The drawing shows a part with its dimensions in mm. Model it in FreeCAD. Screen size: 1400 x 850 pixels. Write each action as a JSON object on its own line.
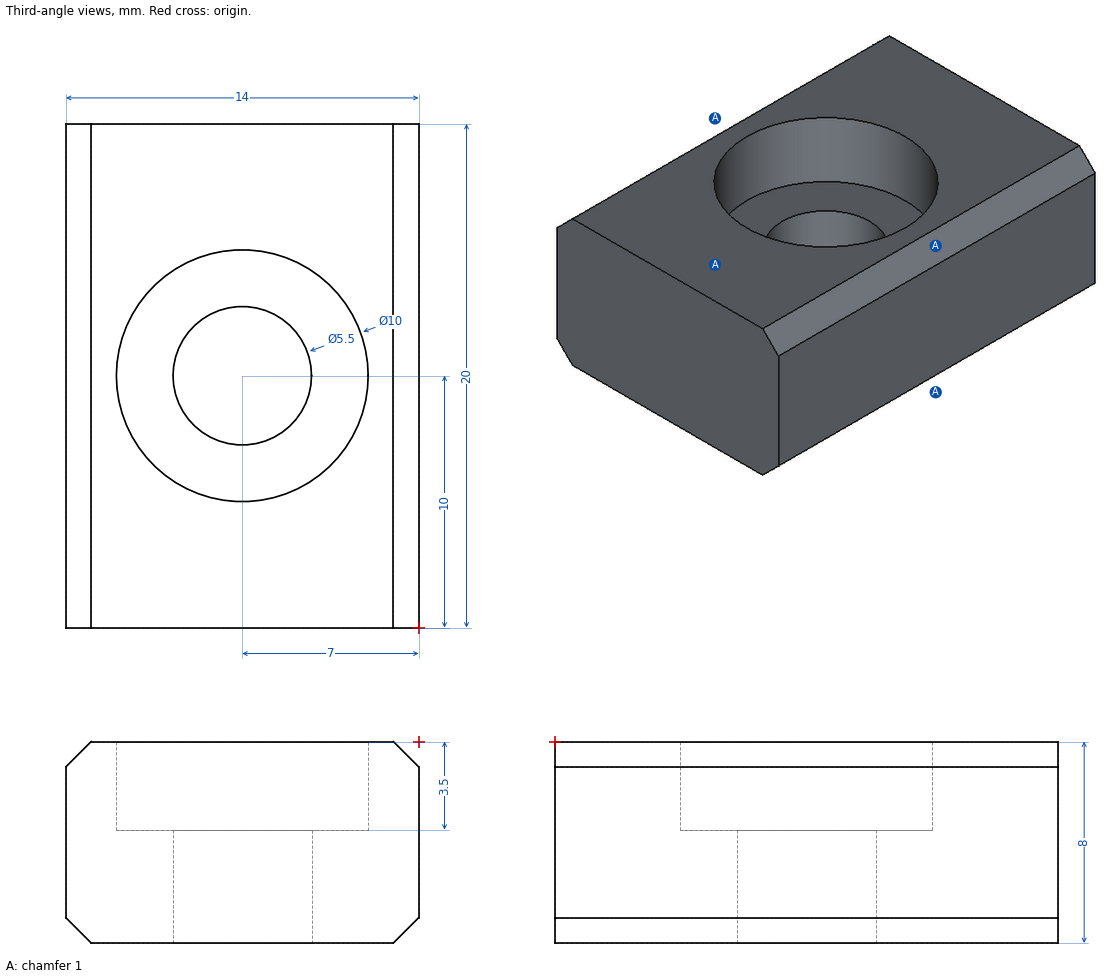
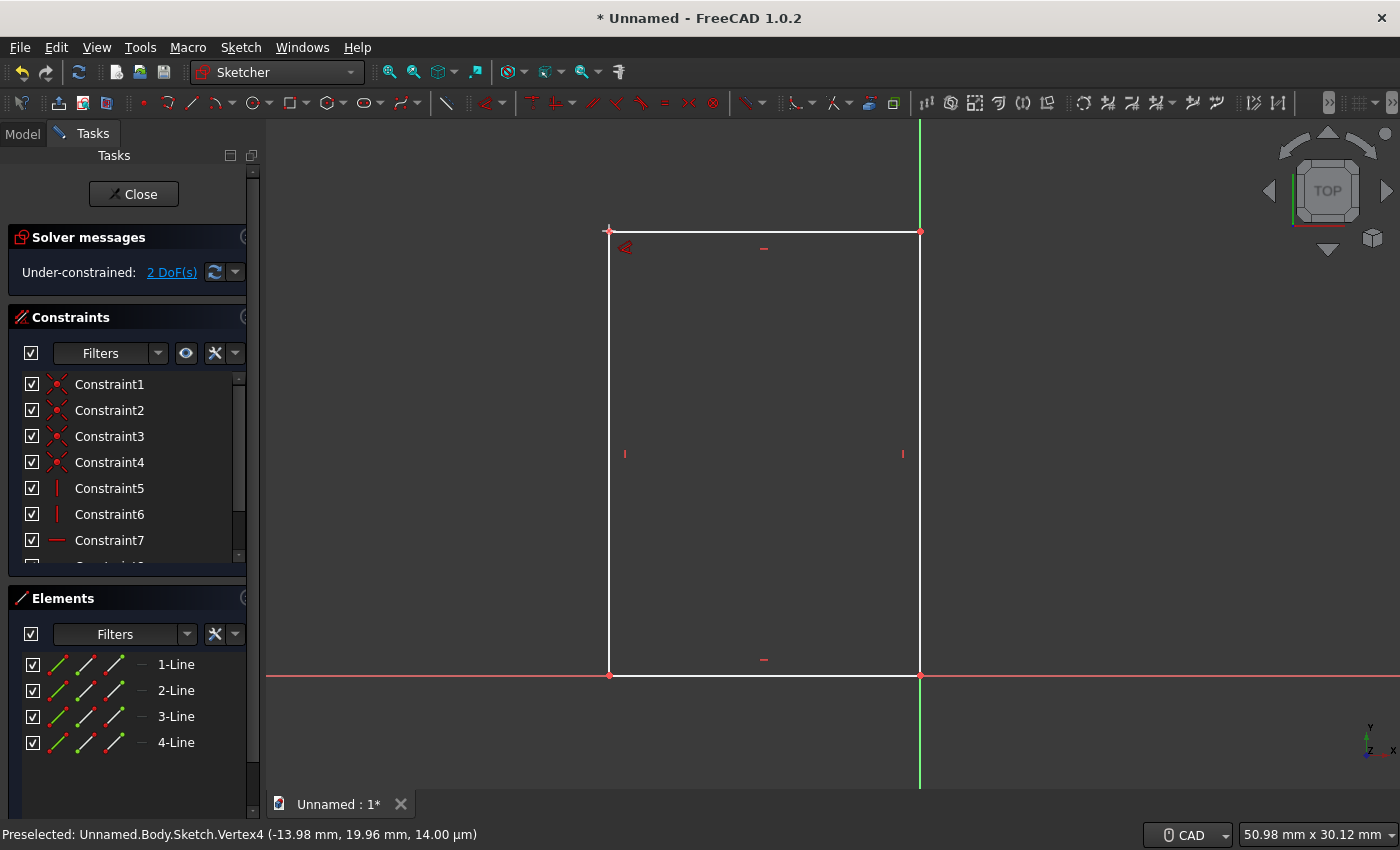
{"action": "left_click", "coordinate": [920, 543]}
{"action": "left_click", "coordinate": [954, 454]}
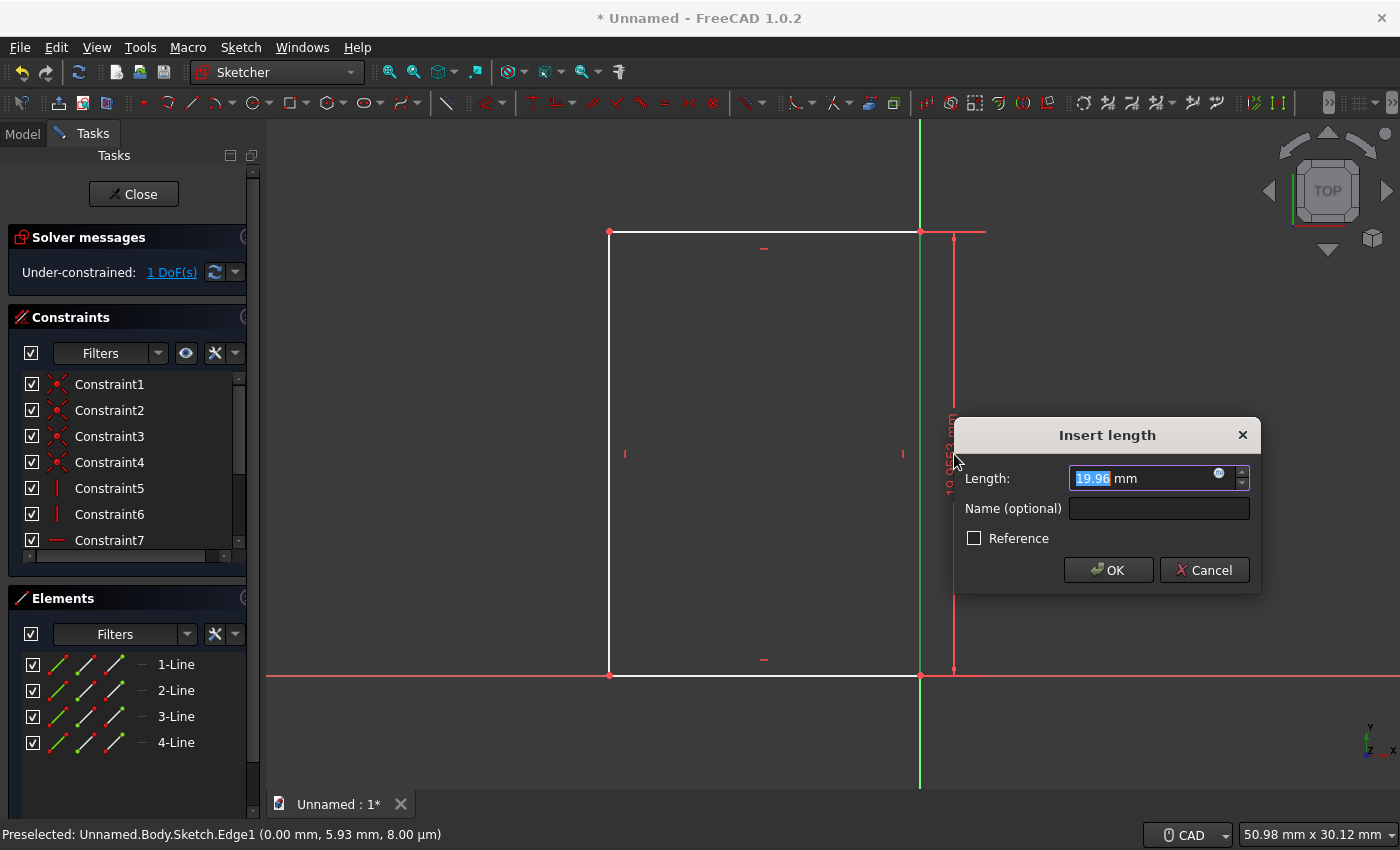
{"action": "type", "text": "20"}
{"action": "key", "text": "Return"}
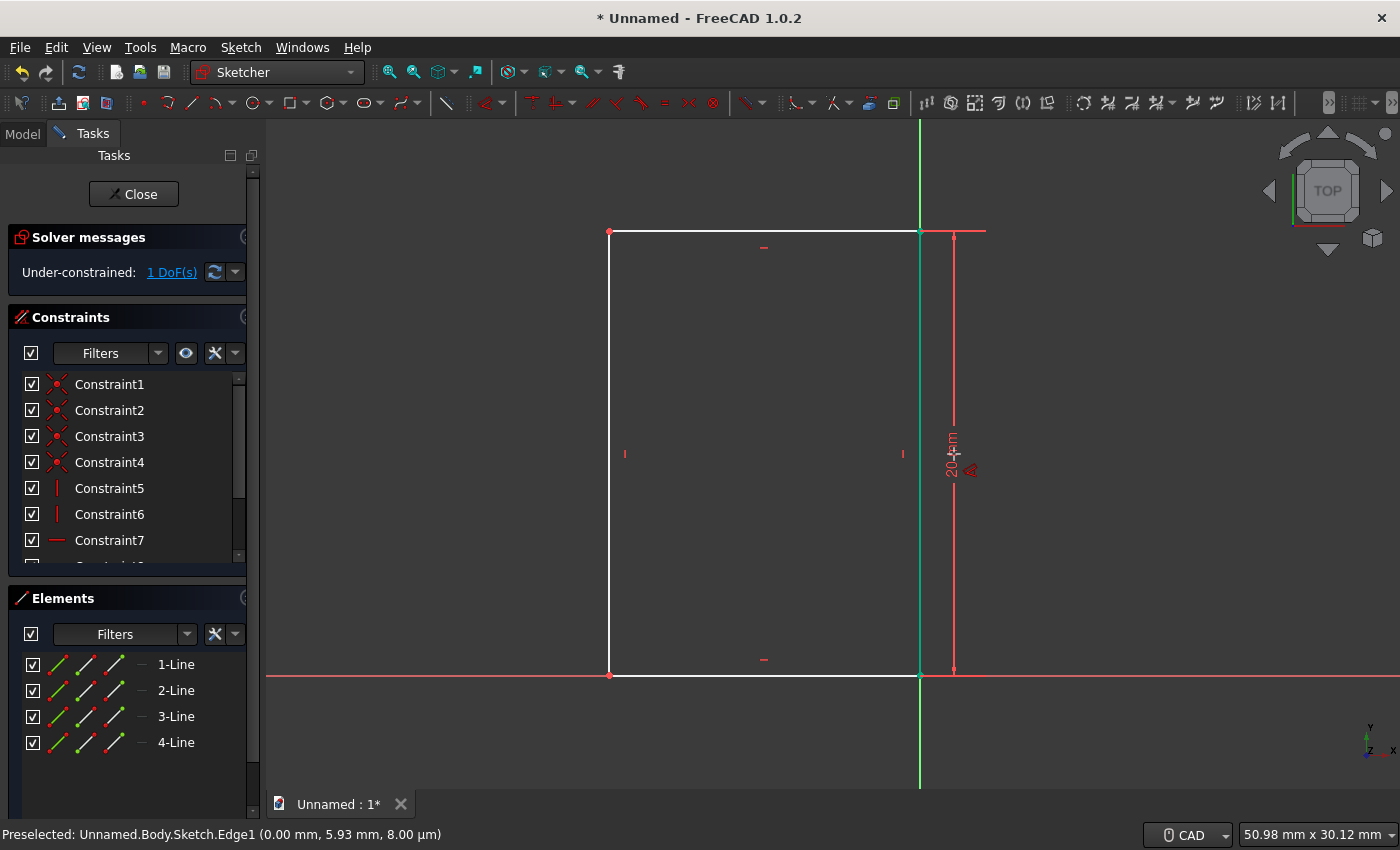
{"action": "left_click", "coordinate": [827, 231]}
{"action": "left_click", "coordinate": [765, 197]}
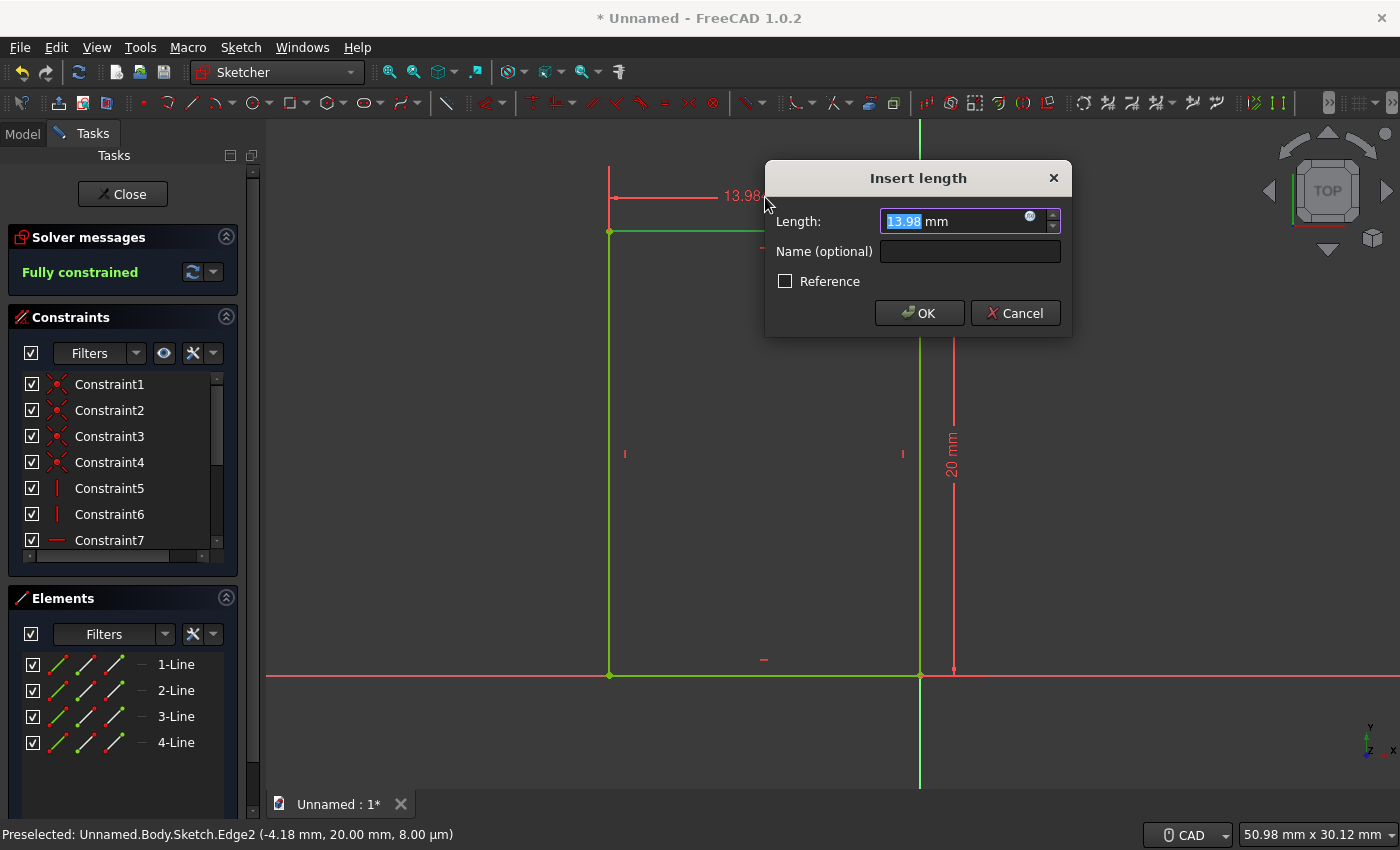
{"action": "type", "text": "14"}
{"action": "key", "text": "Return"}
{"action": "key", "text": "Escape"}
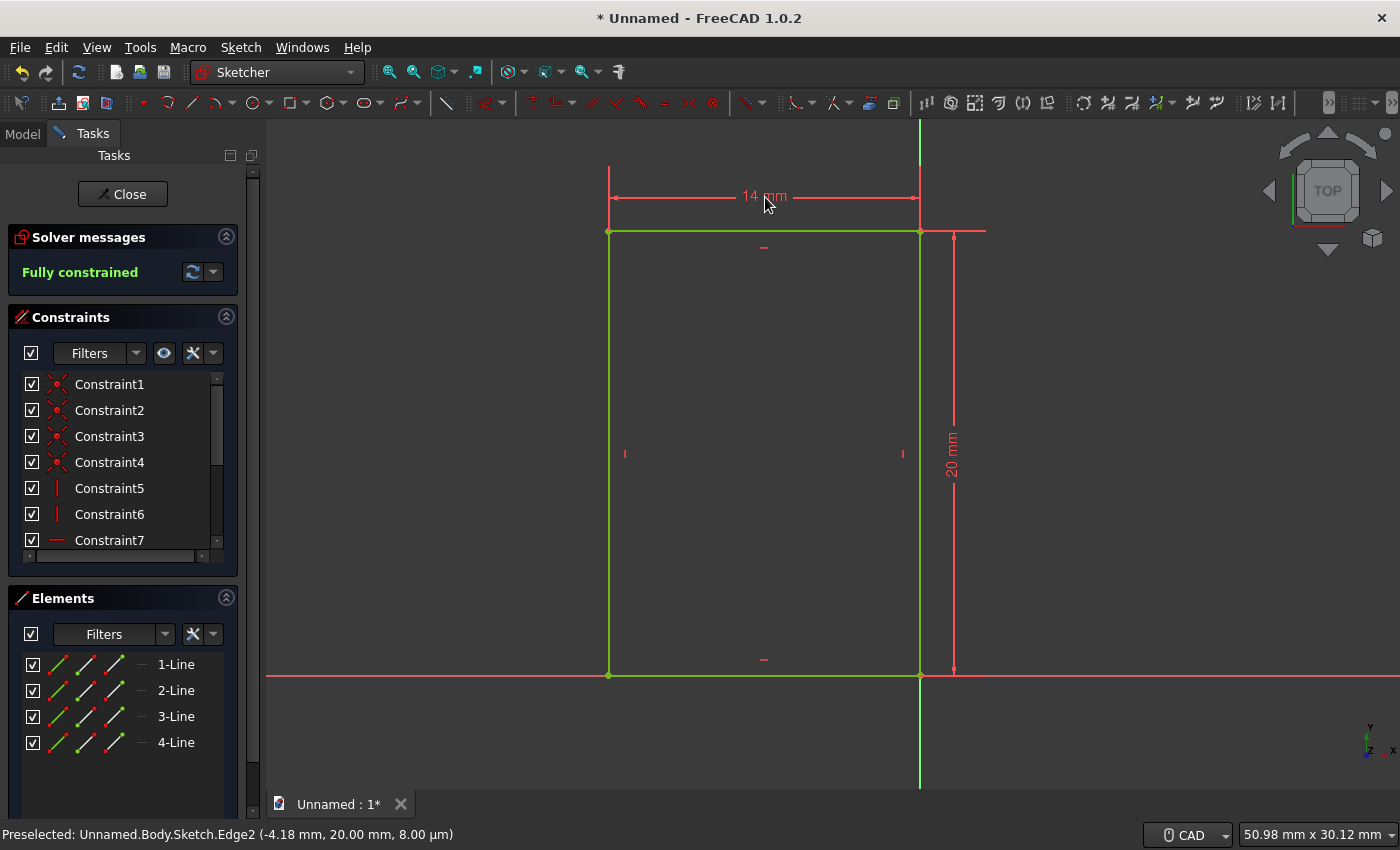
{"action": "left_click", "coordinate": [123, 194]}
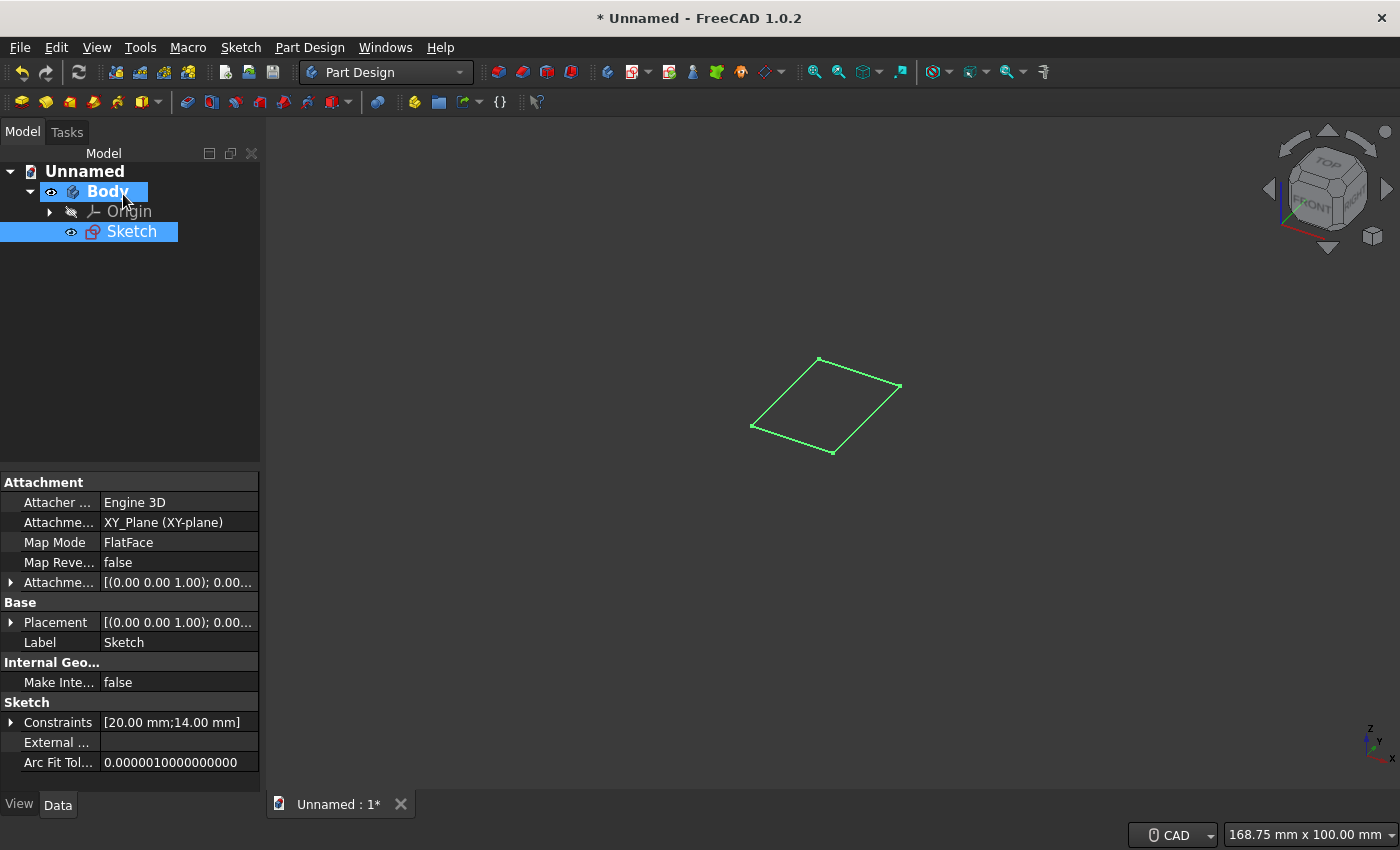
{"action": "left_click", "coordinate": [22, 102]}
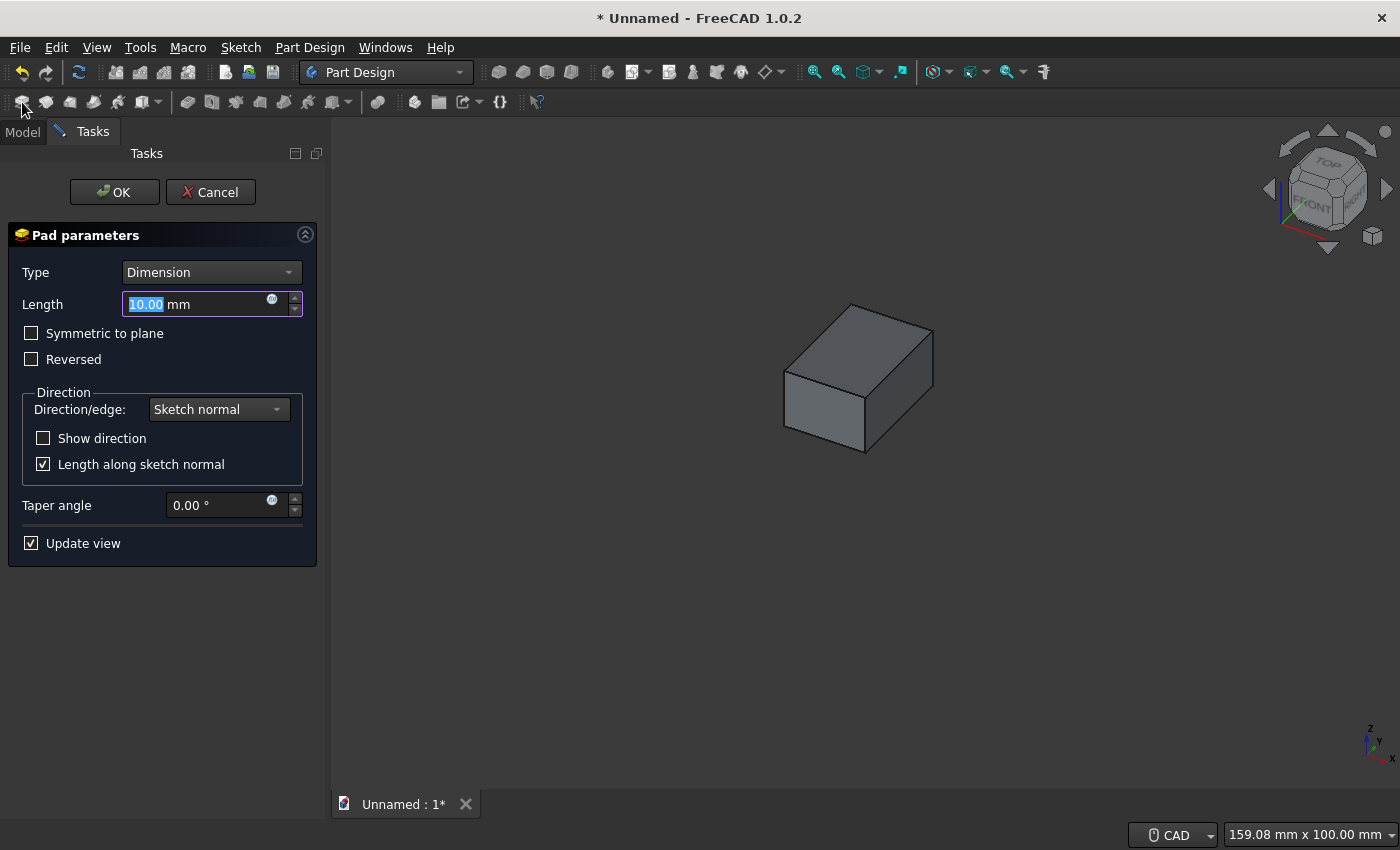
{"action": "type", "text": "8"}
{"action": "key", "text": "Tab"}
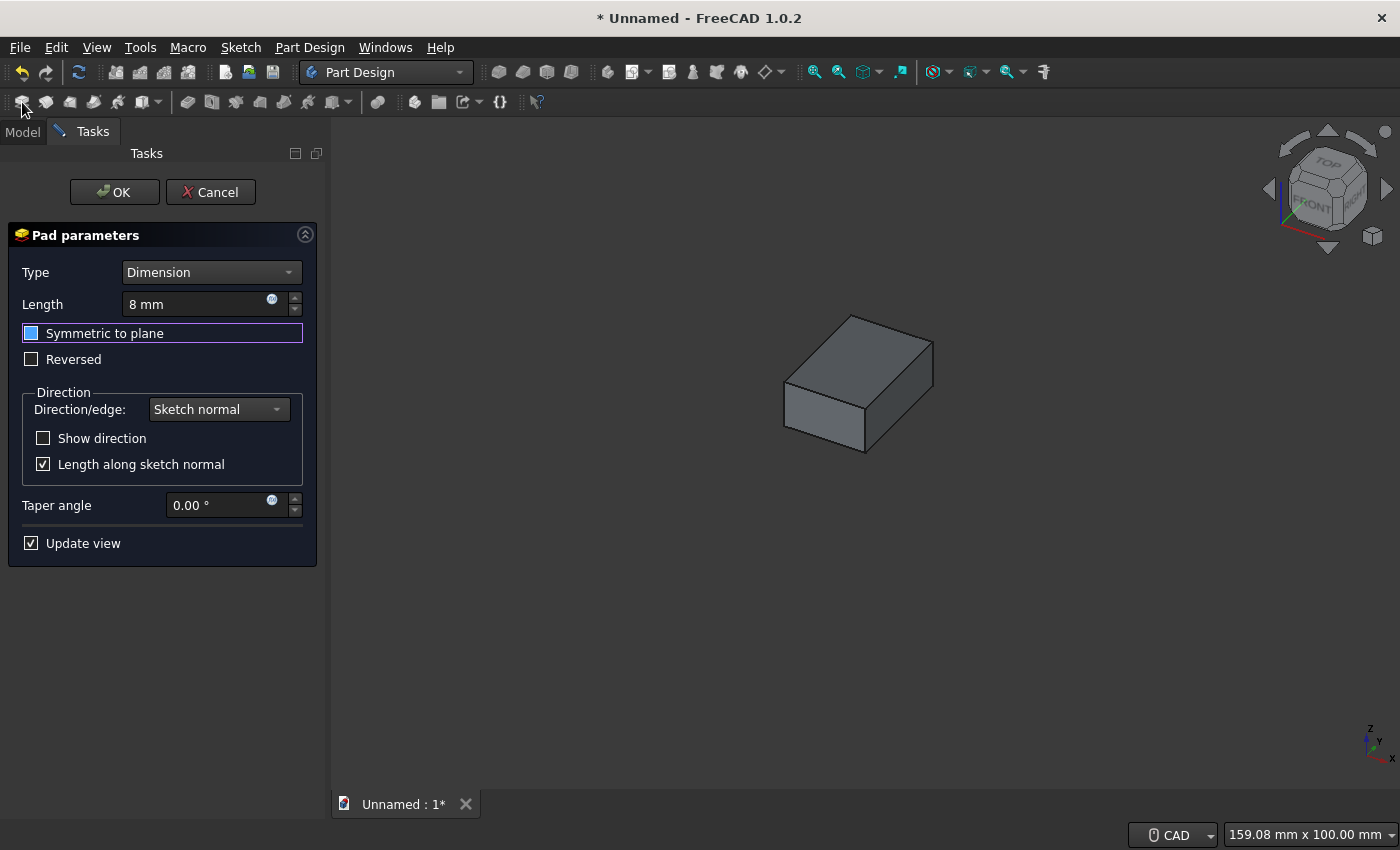
{"action": "left_click", "coordinate": [30, 359]}